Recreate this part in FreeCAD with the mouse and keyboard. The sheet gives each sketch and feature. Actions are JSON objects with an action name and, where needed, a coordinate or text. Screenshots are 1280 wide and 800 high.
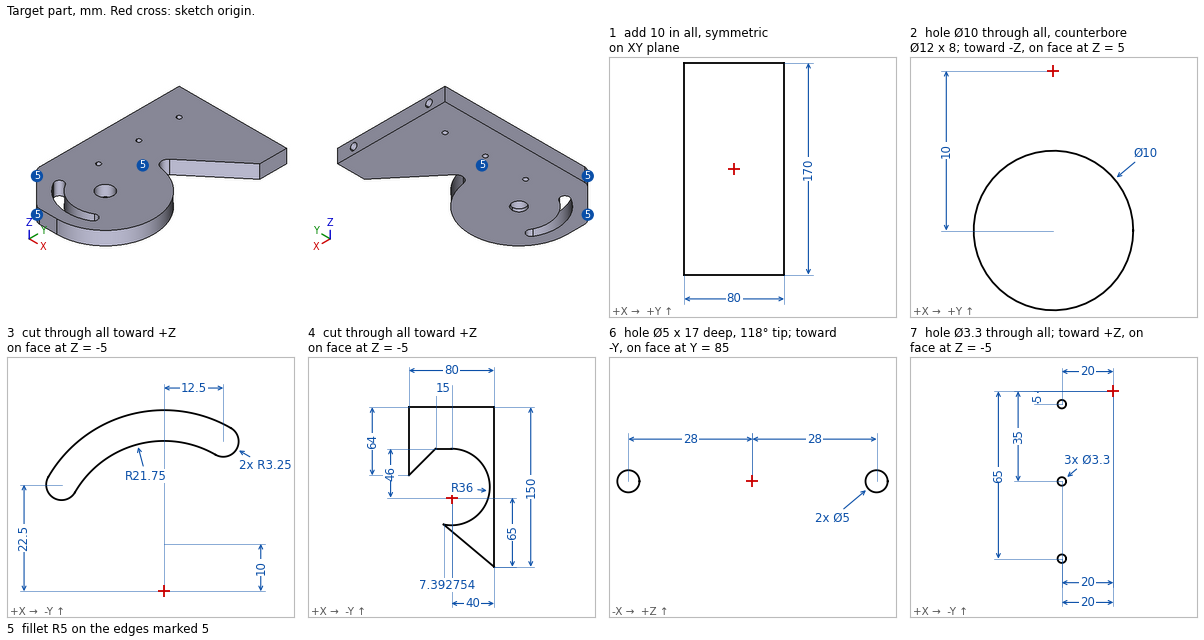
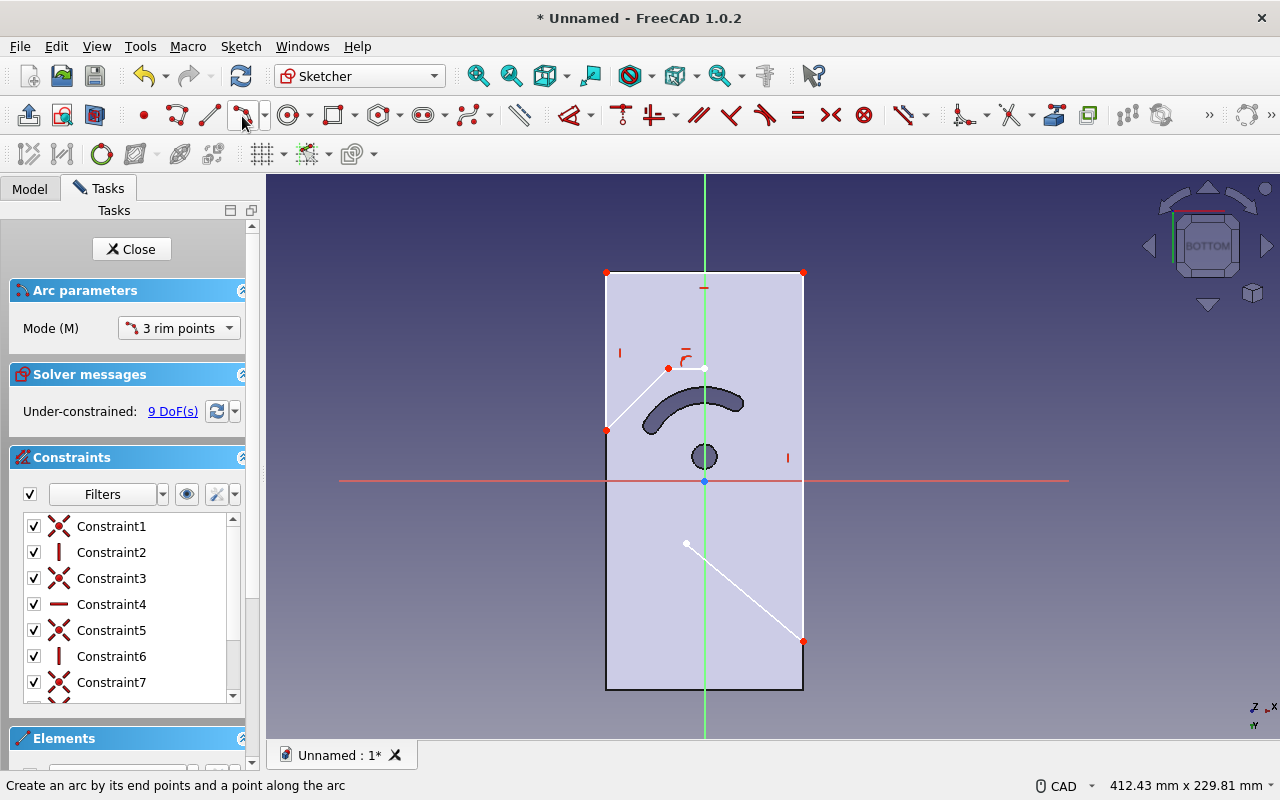
{"action": "left_click", "coordinate": [705, 369]}
{"action": "left_click", "coordinate": [686, 544]}
{"action": "left_click", "coordinate": [768, 518]}
{"action": "key", "text": "Escape"}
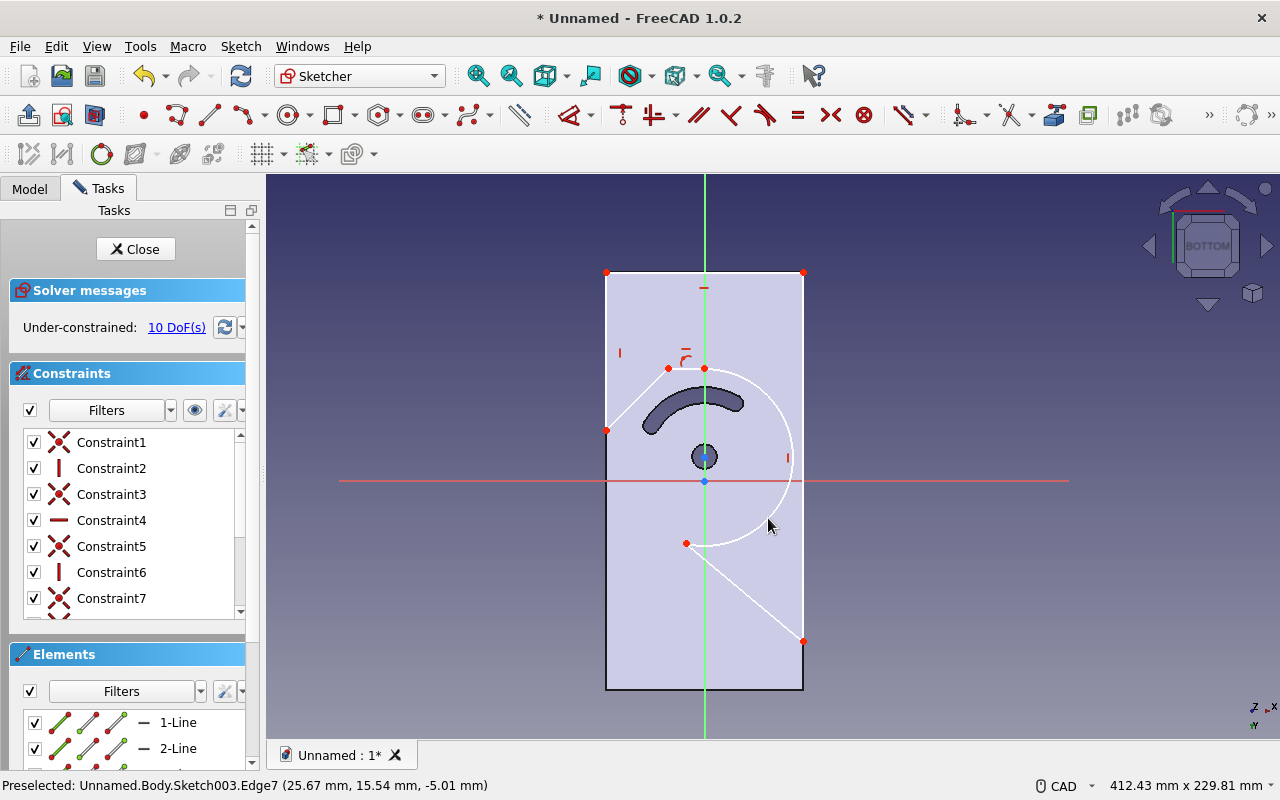
{"action": "left_click", "coordinate": [704, 457]}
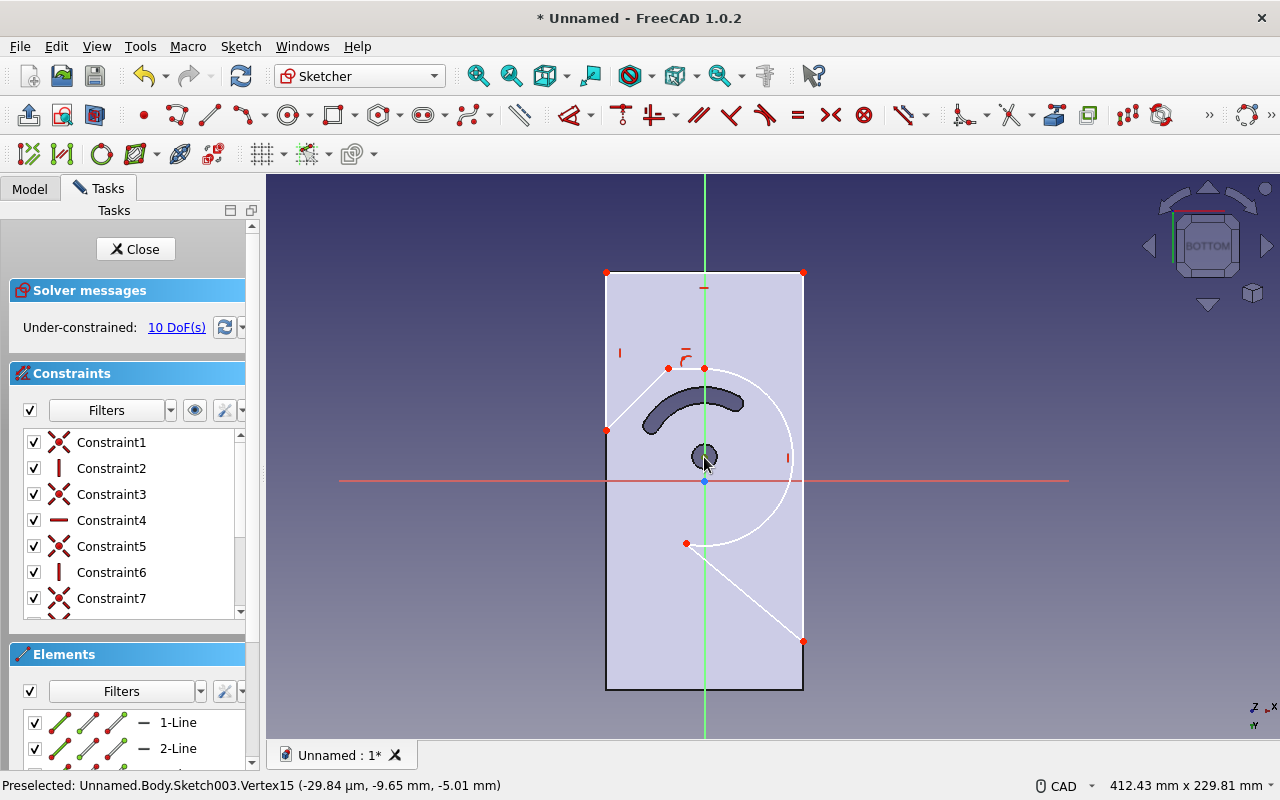
{"action": "left_click", "coordinate": [705, 675]}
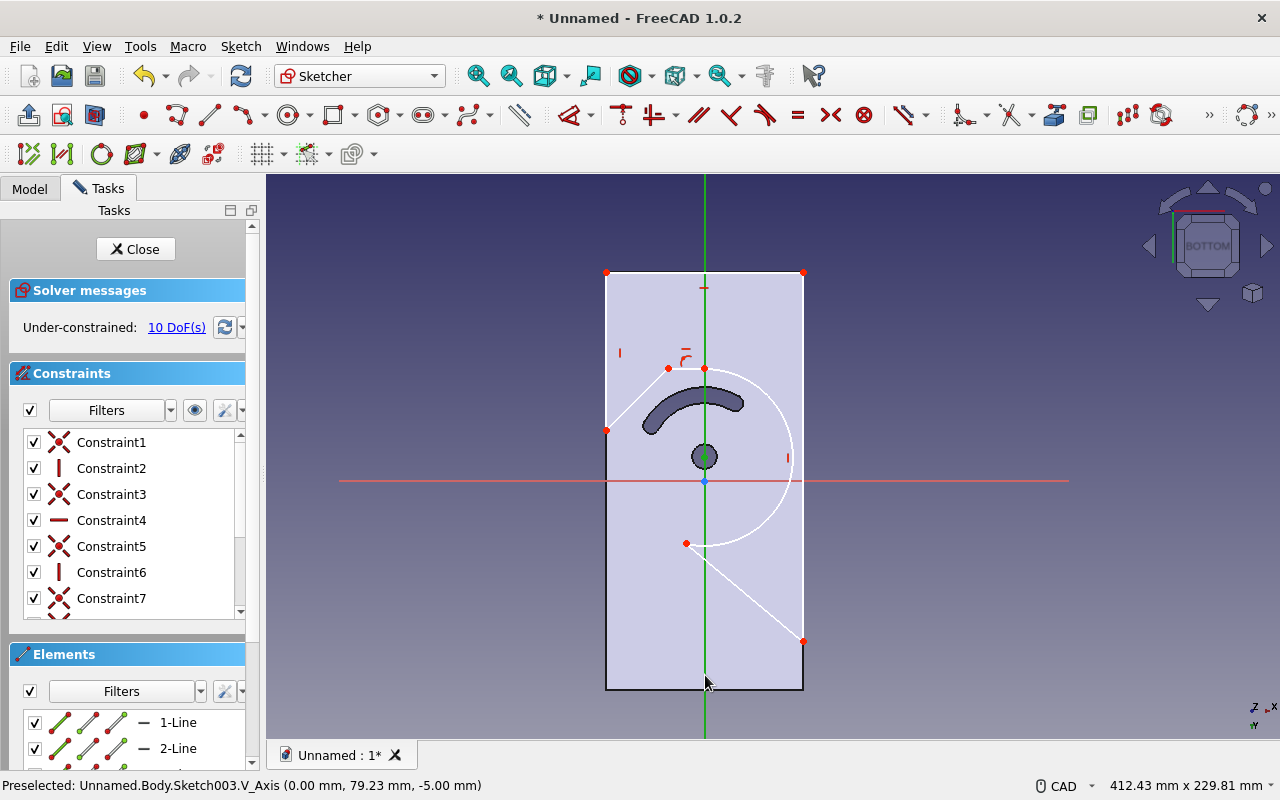
{"action": "key", "text": "c"}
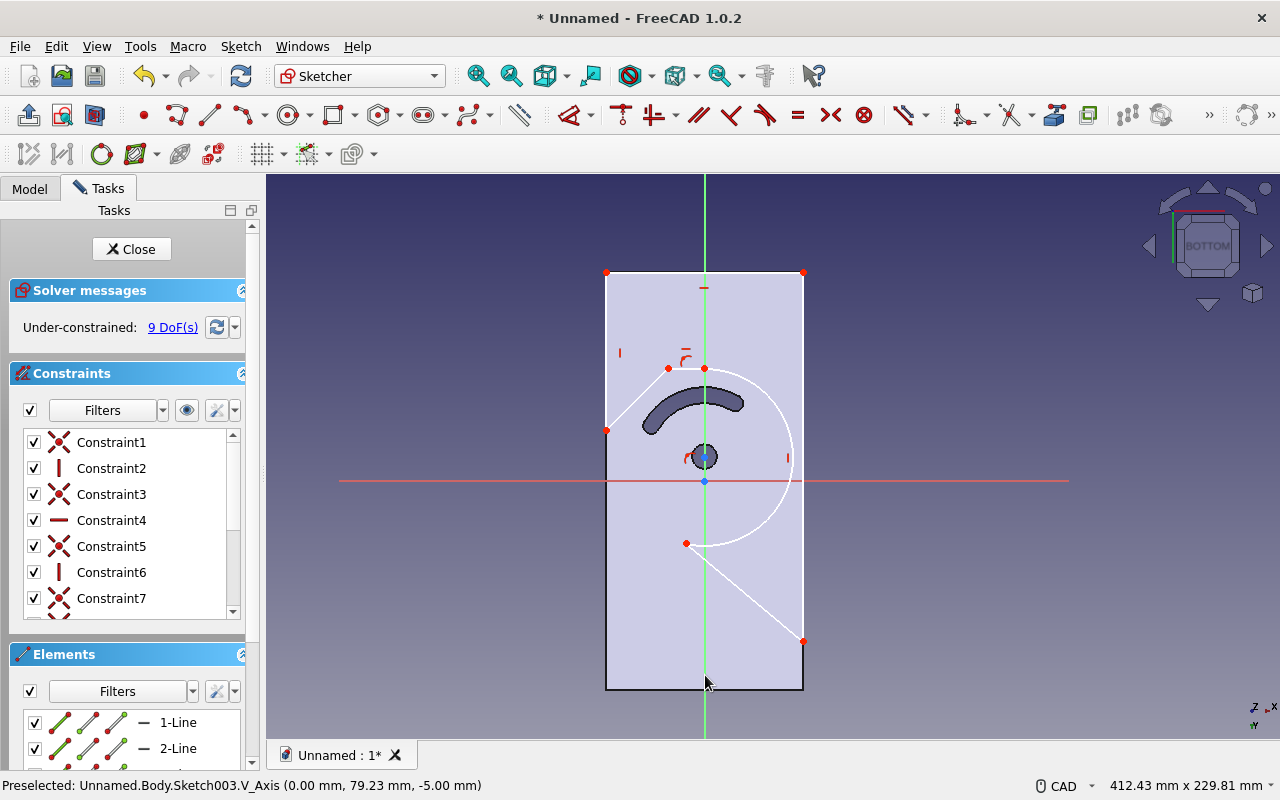
{"action": "key", "text": "d"}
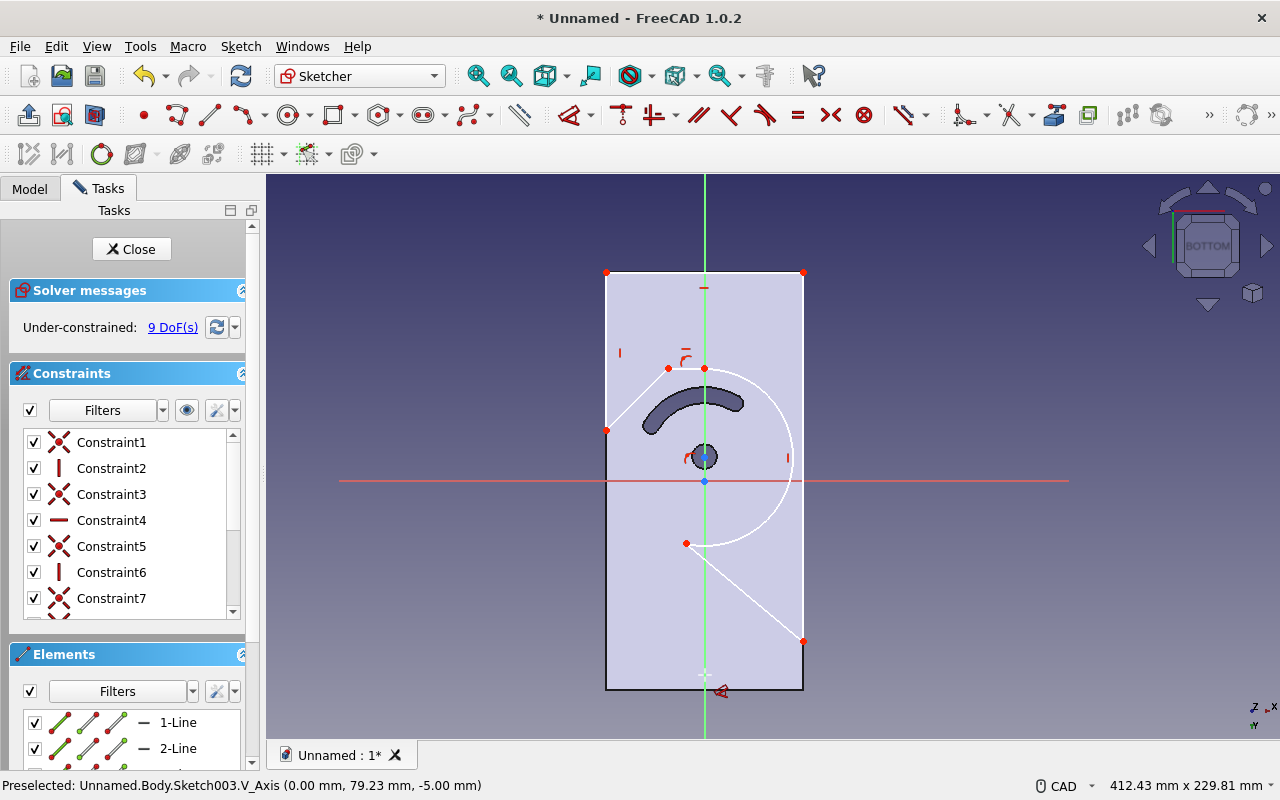
{"action": "left_click", "coordinate": [768, 519]}
{"action": "left_click", "coordinate": [681, 576]}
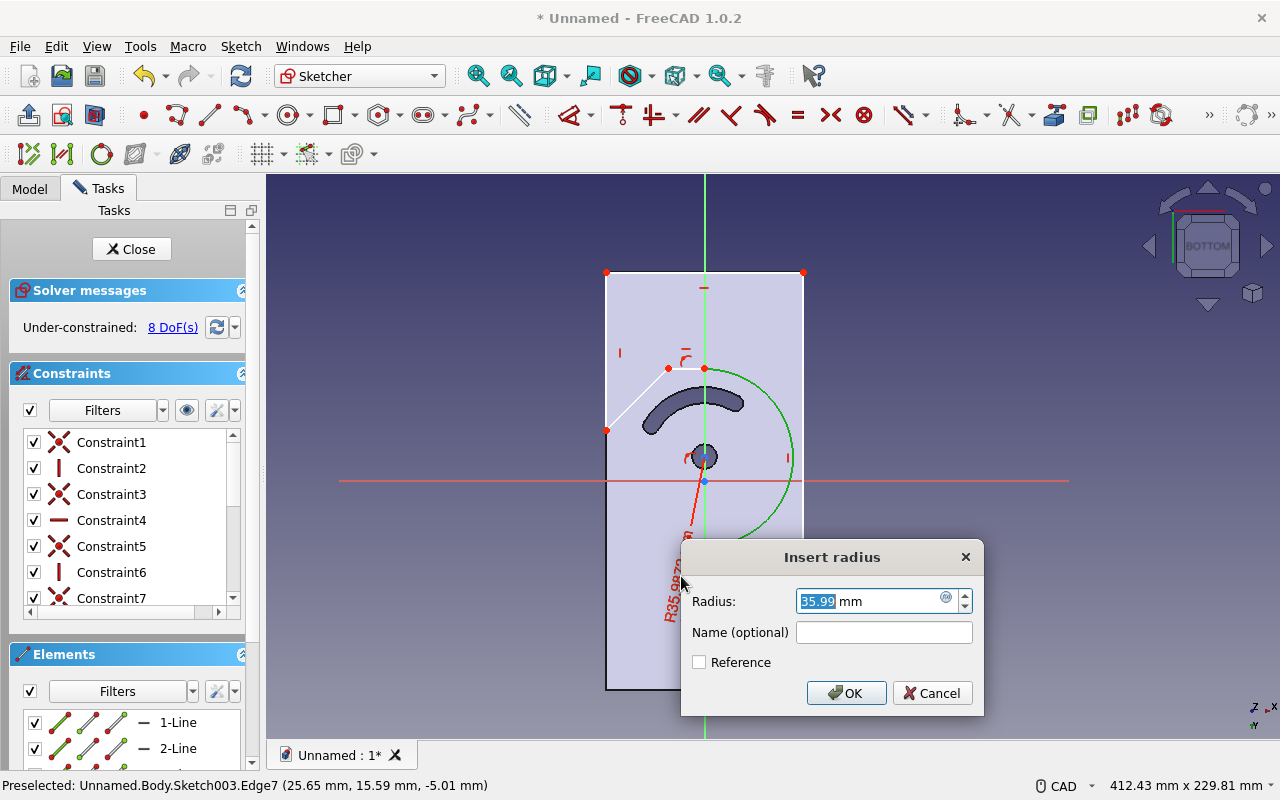
{"action": "type", "text": "36"}
{"action": "key", "text": "Return"}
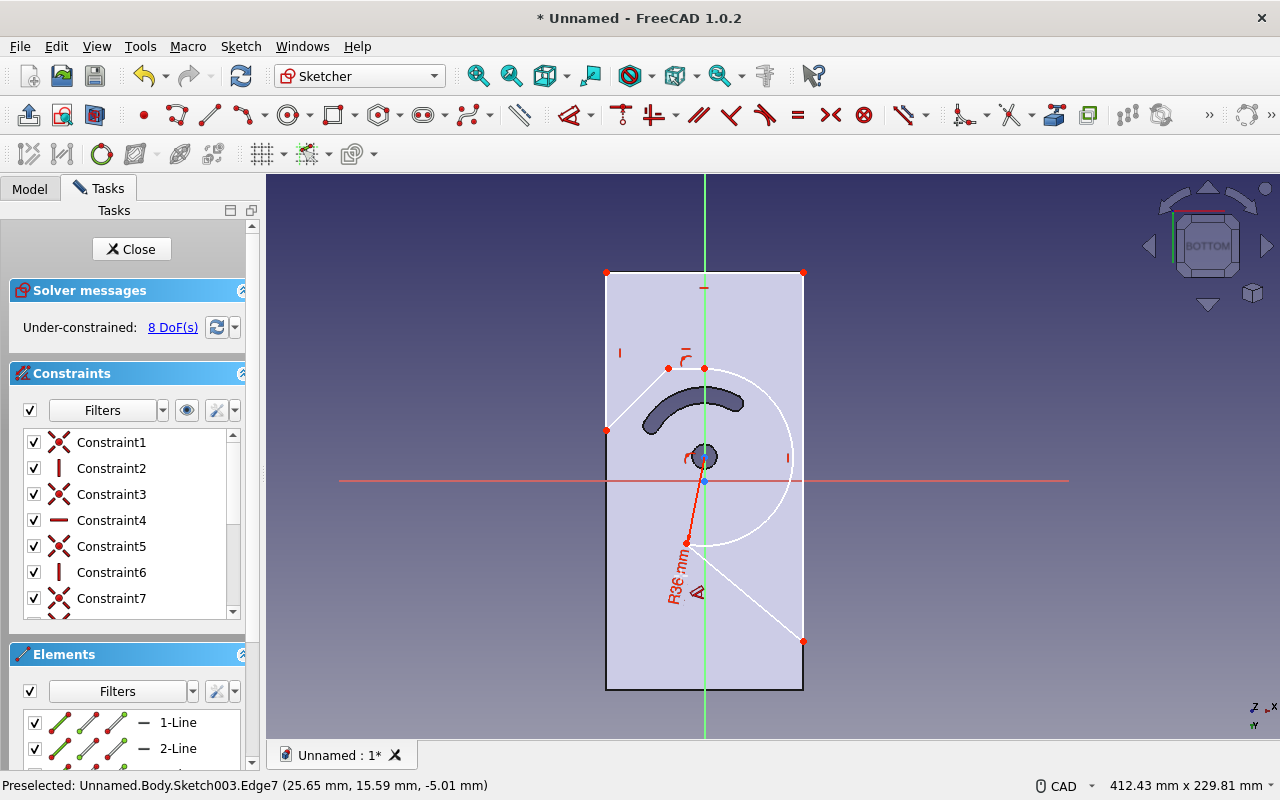
{"action": "left_click", "coordinate": [744, 273]}
{"action": "left_click", "coordinate": [659, 239]}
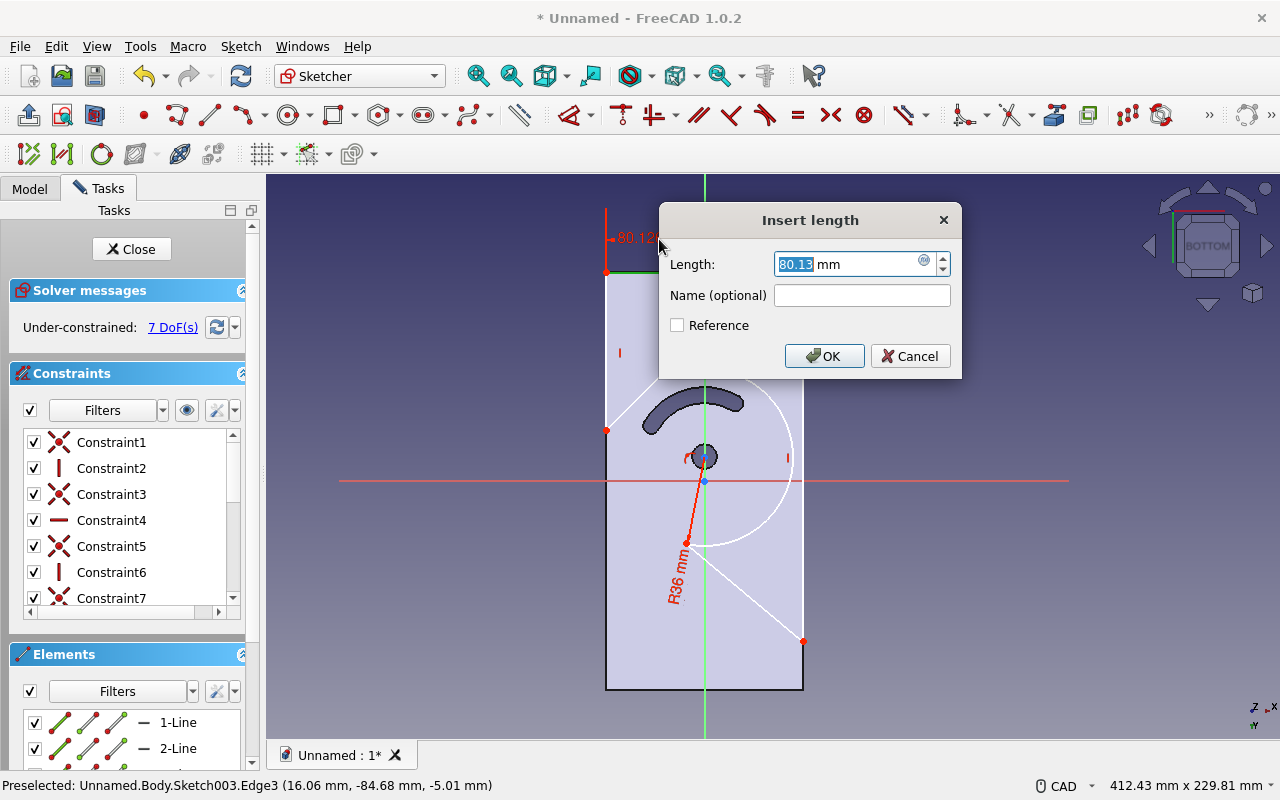
{"action": "type", "text": "80"}
{"action": "key", "text": "Return"}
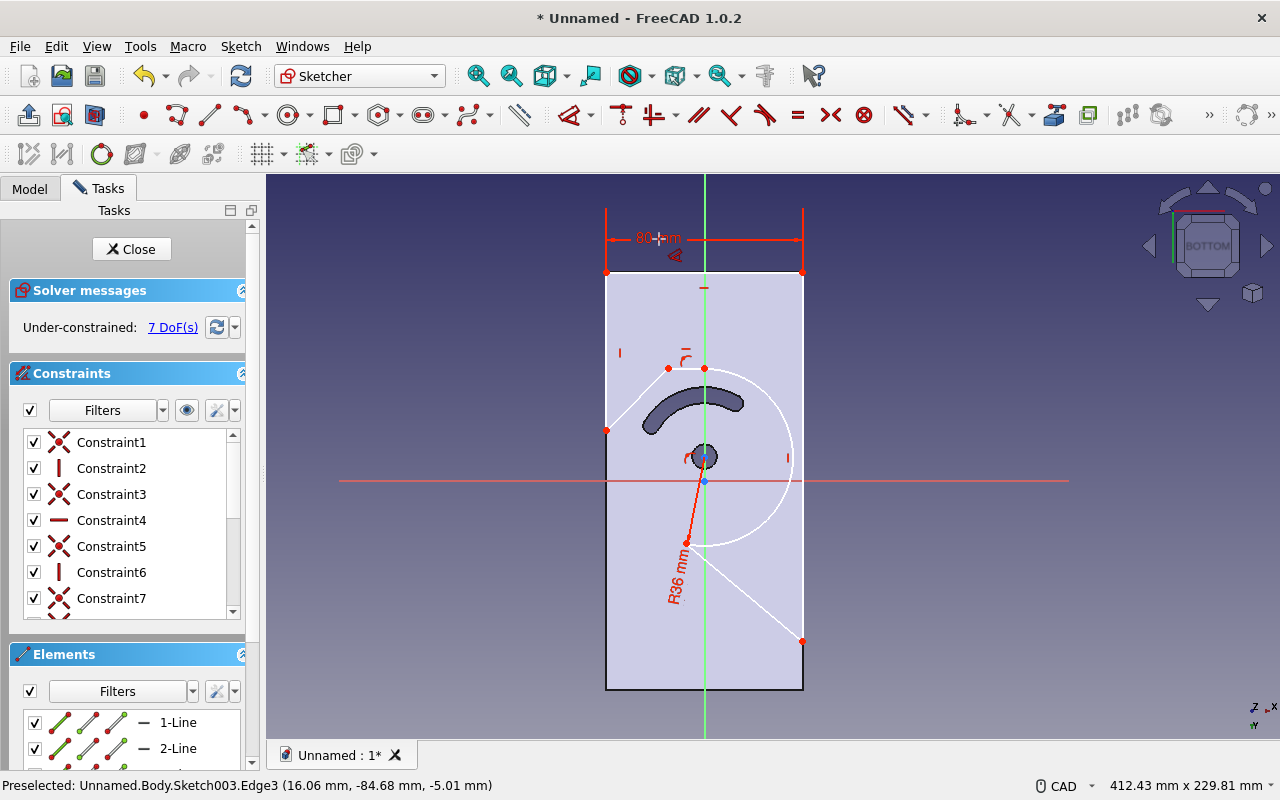
{"action": "left_click", "coordinate": [606, 320]}
{"action": "left_click", "coordinate": [572, 352]}